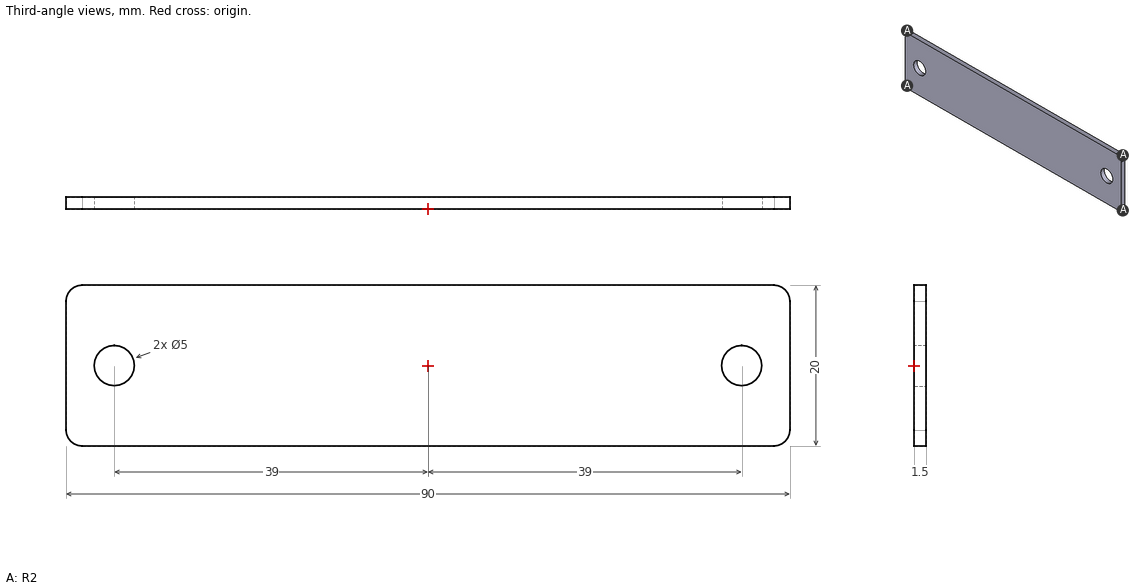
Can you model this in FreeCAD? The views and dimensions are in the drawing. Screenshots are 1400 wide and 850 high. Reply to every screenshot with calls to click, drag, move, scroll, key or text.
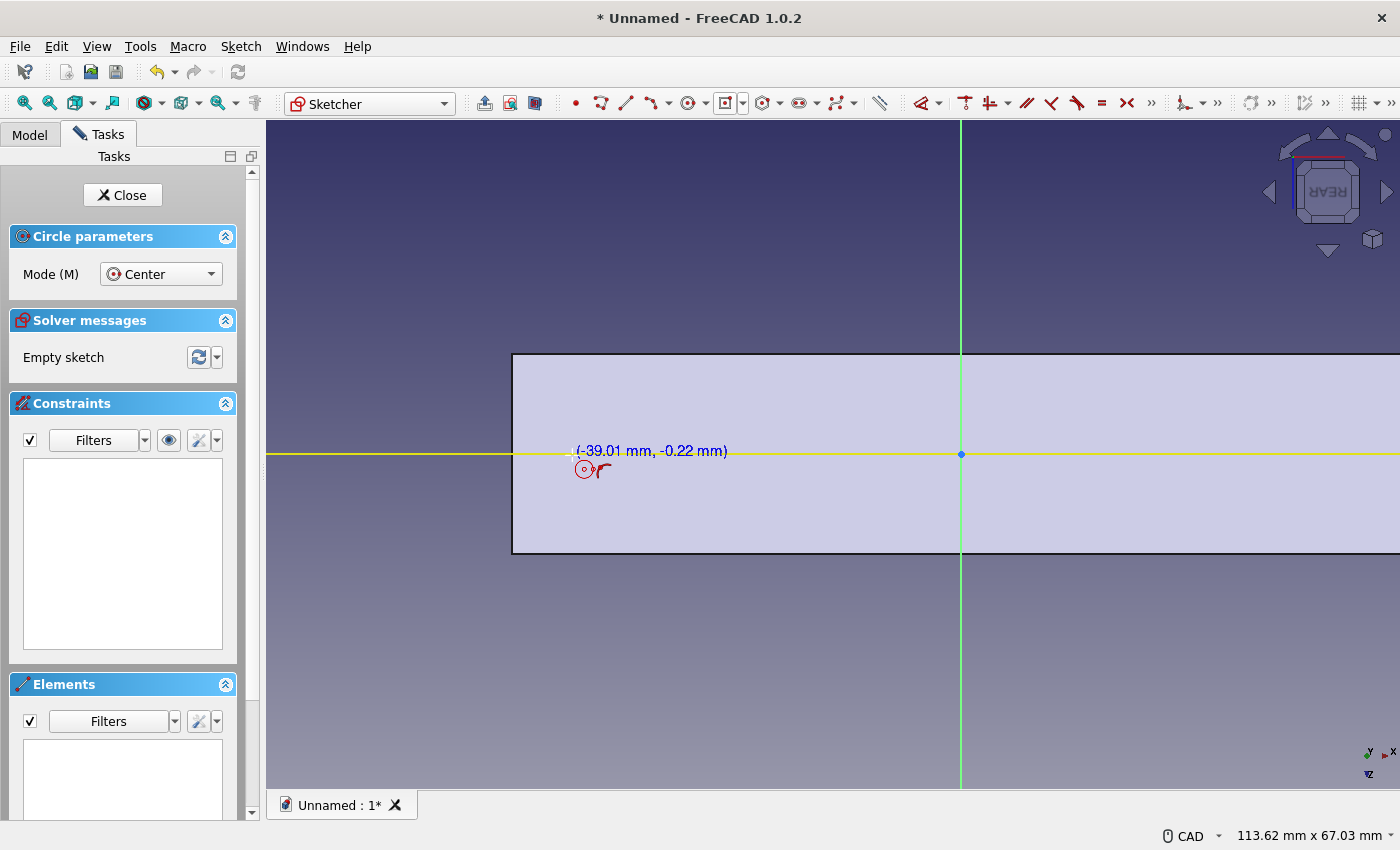
click(572, 454)
move(590, 436)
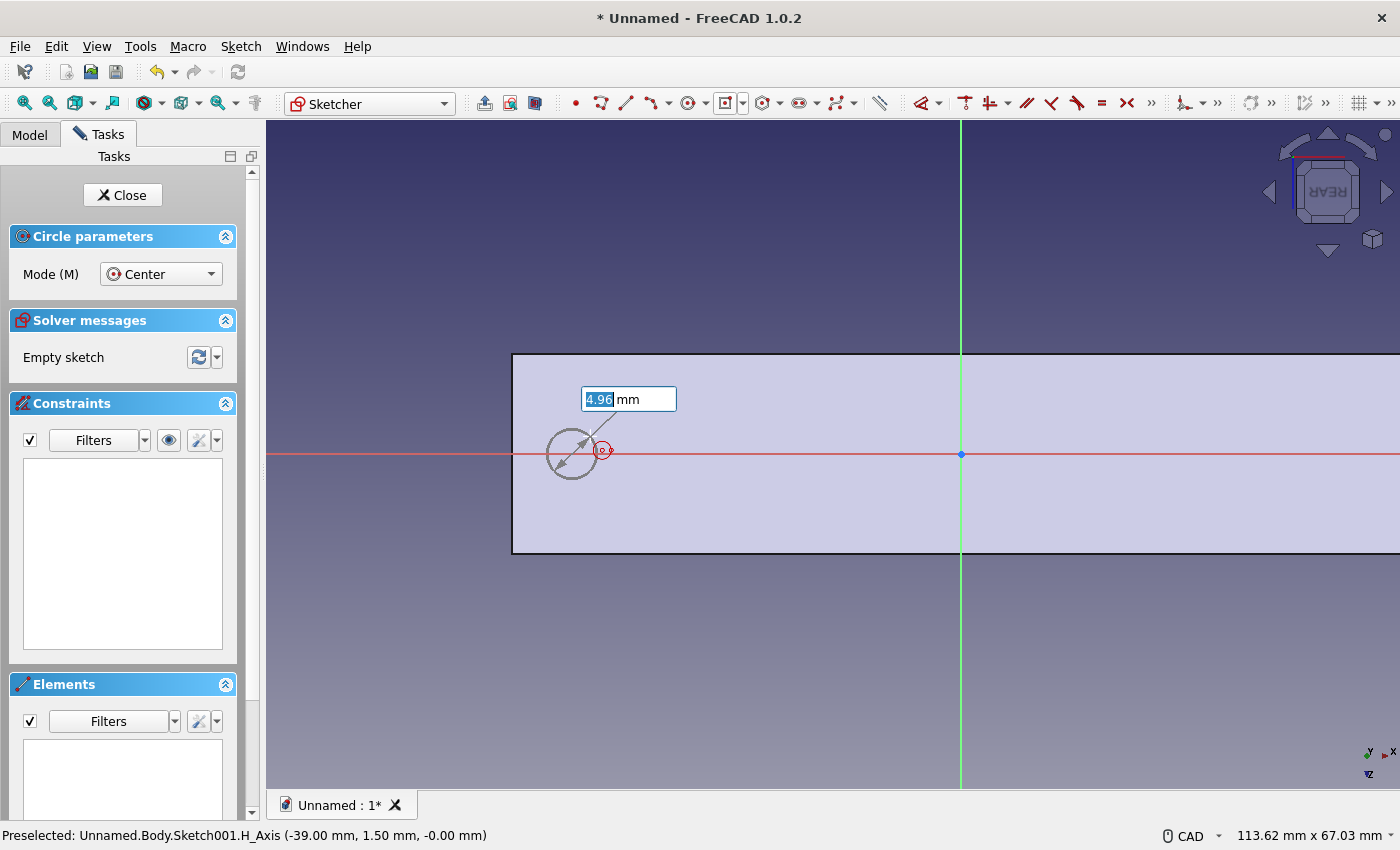
text(5)
key(Return)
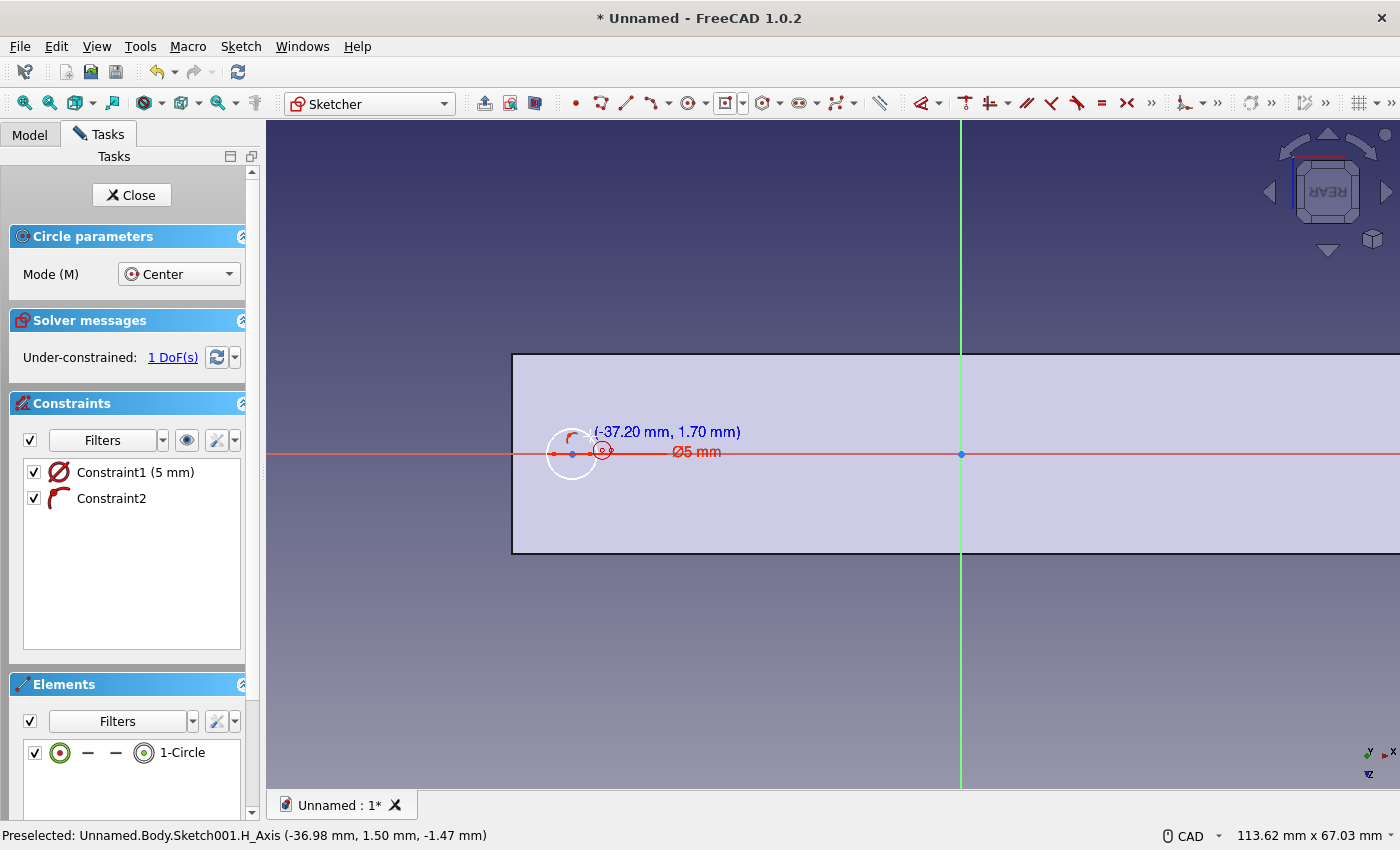
scroll(294, 457, down, 1)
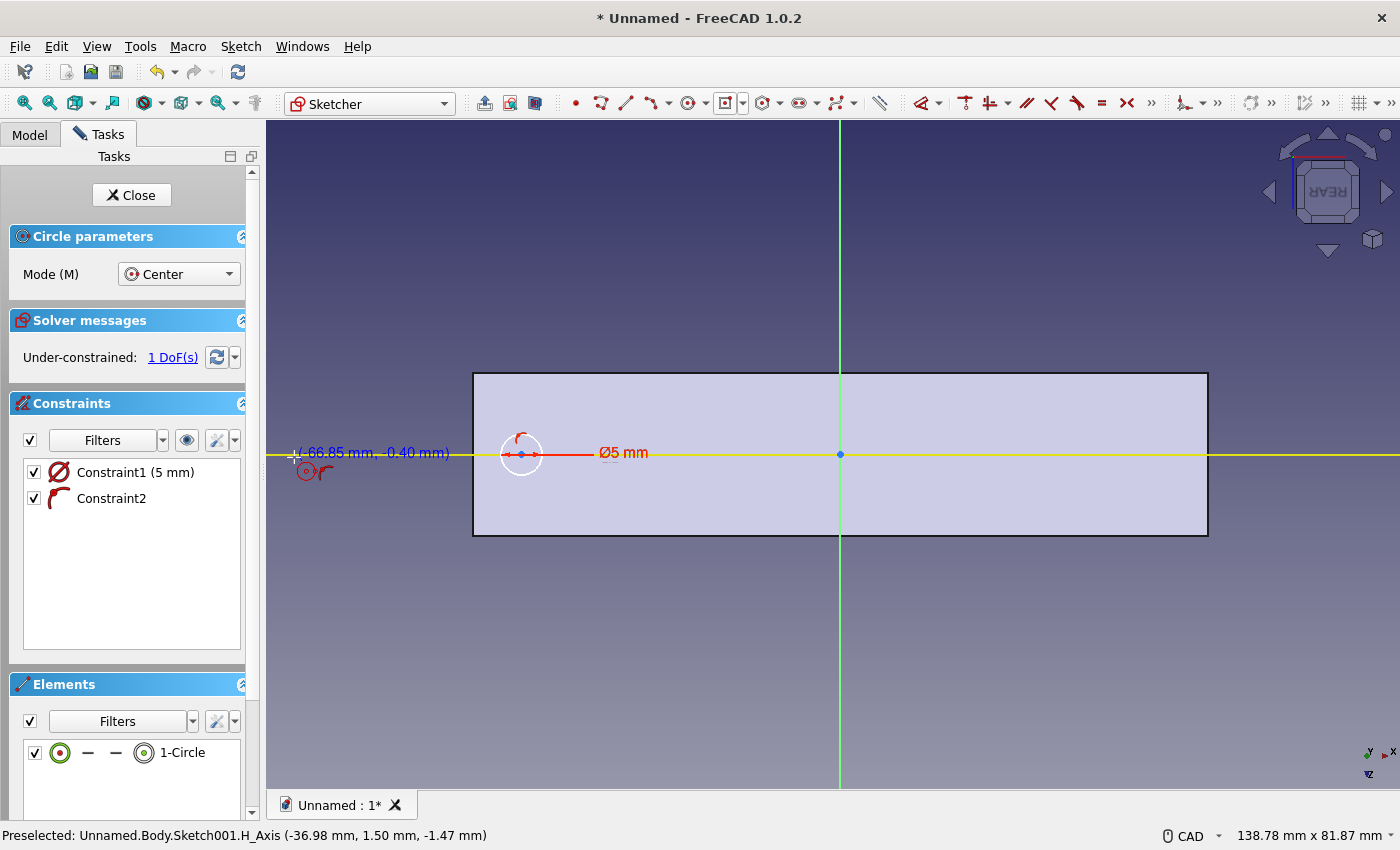
click(1159, 455)
move(1173, 440)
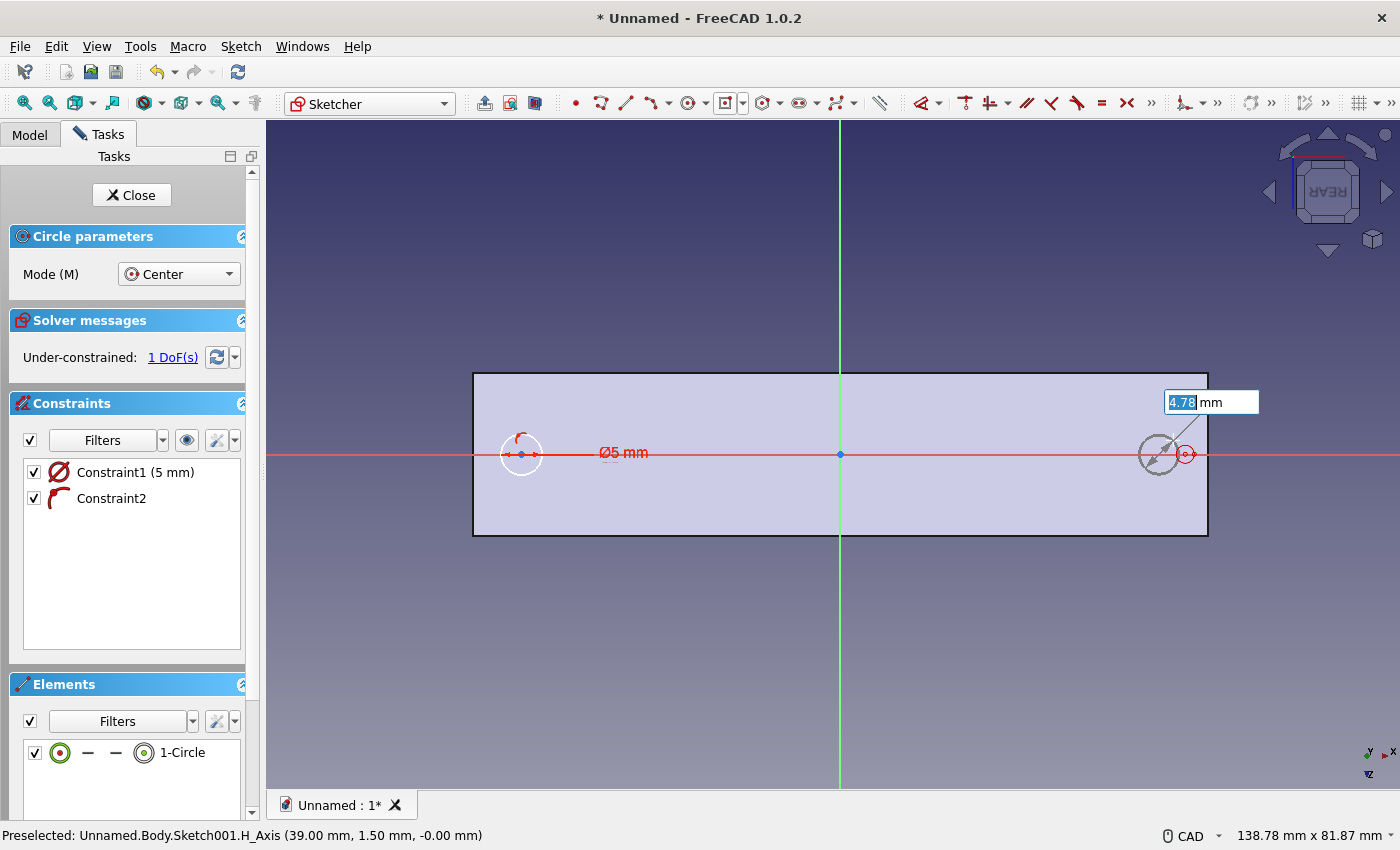
text(5)
key(Return)
key(Escape)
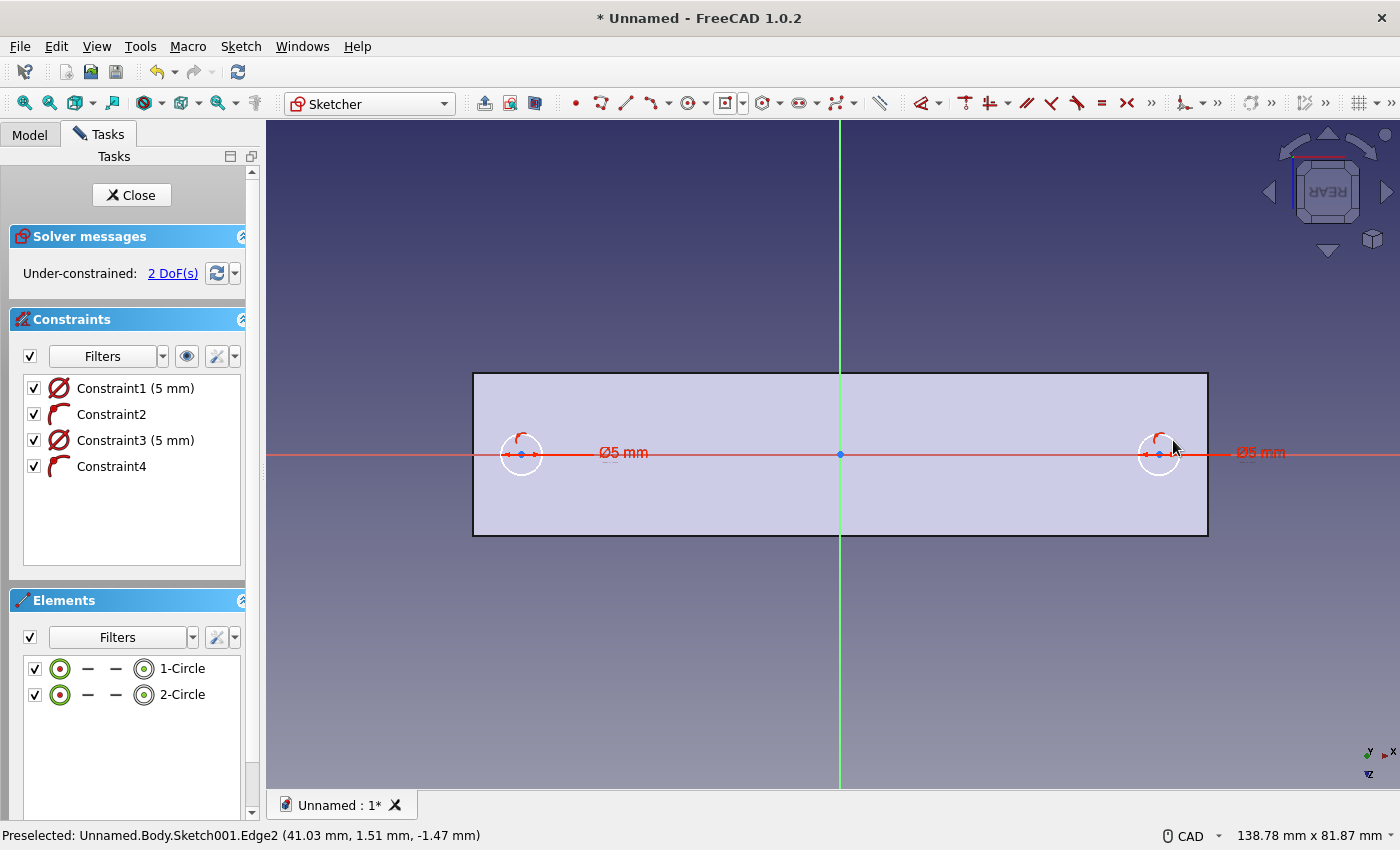
click(920, 104)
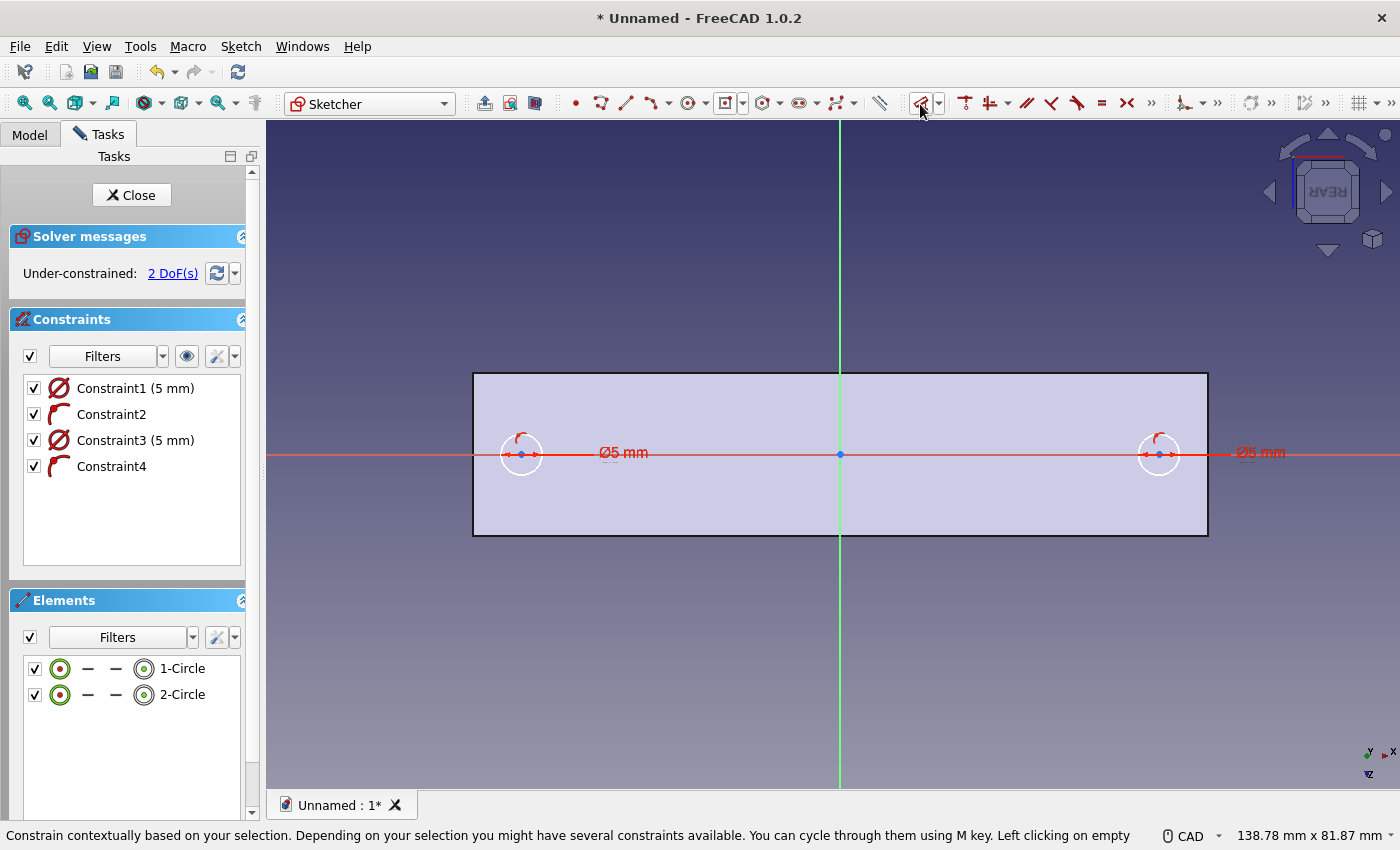
click(522, 455)
click(681, 489)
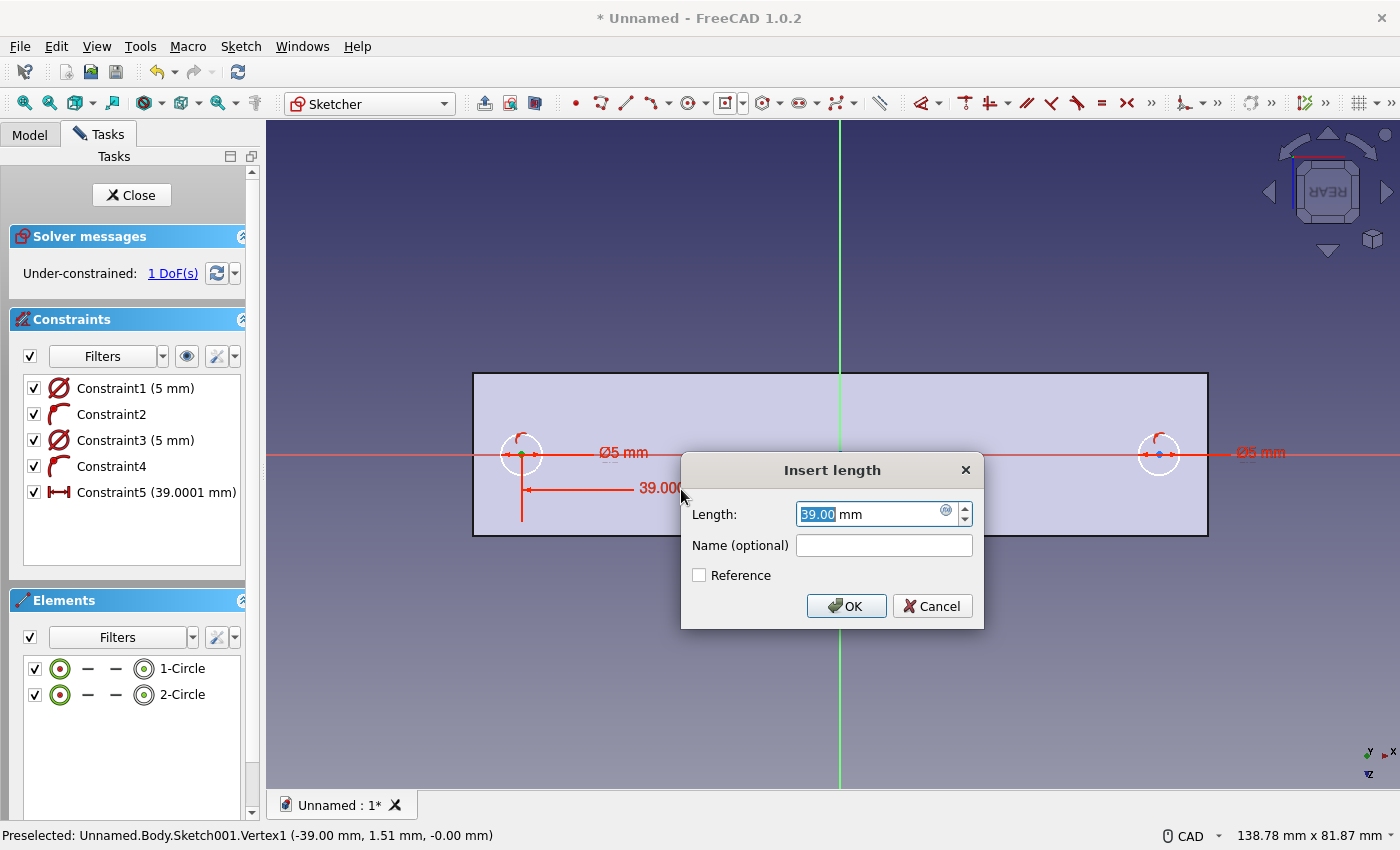
text(39)
key(Return)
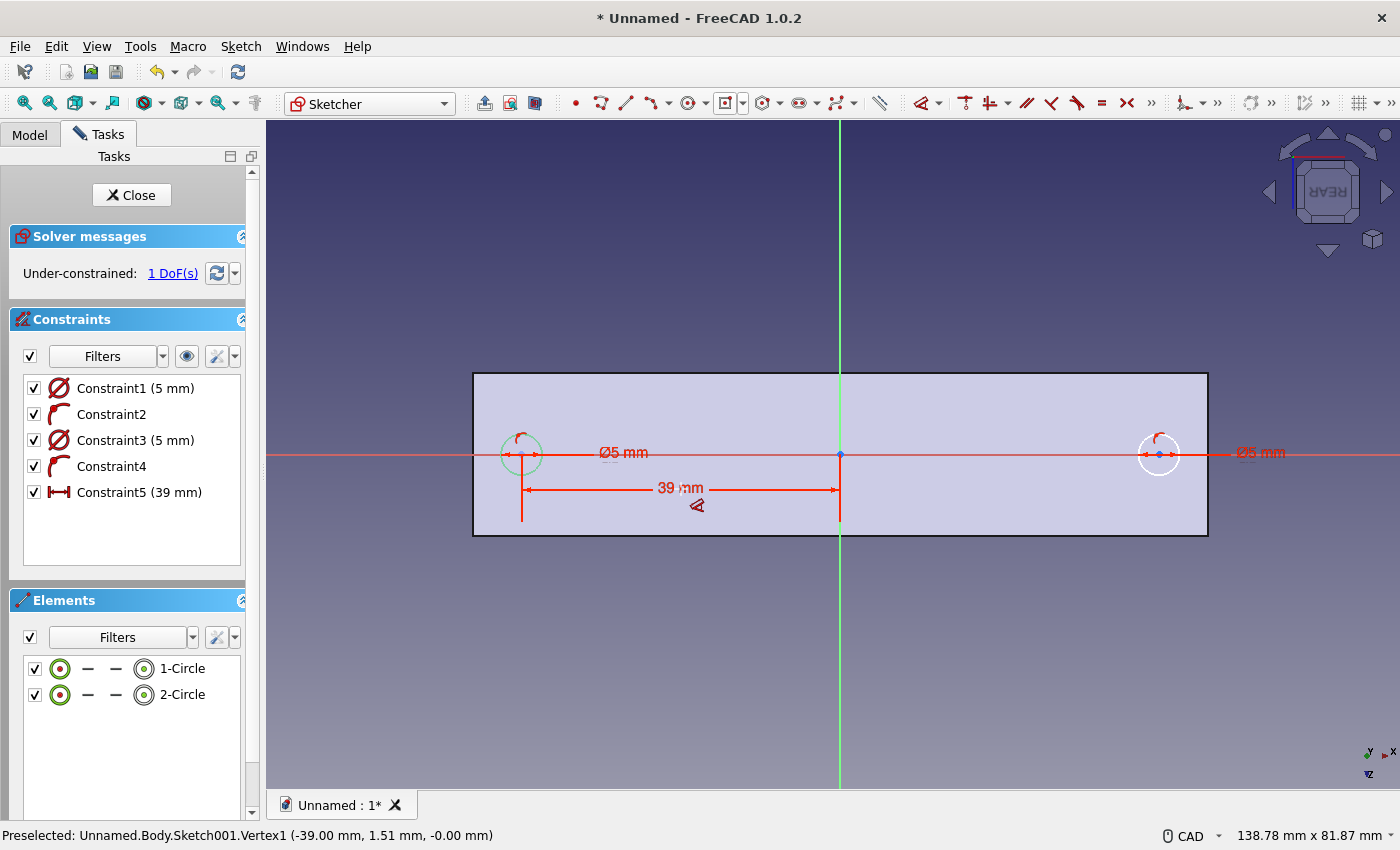
click(1159, 455)
click(1000, 489)